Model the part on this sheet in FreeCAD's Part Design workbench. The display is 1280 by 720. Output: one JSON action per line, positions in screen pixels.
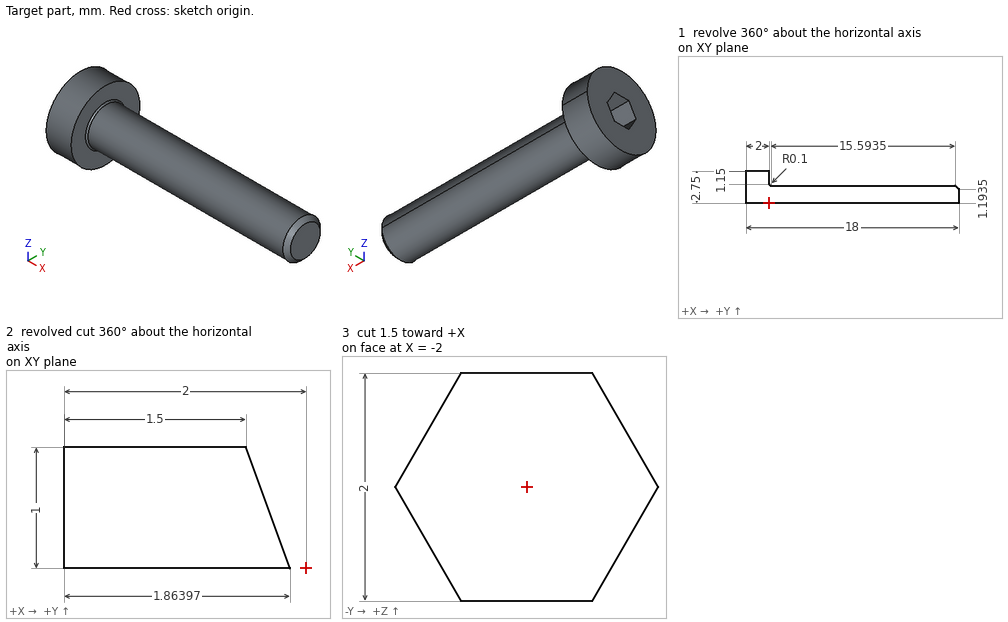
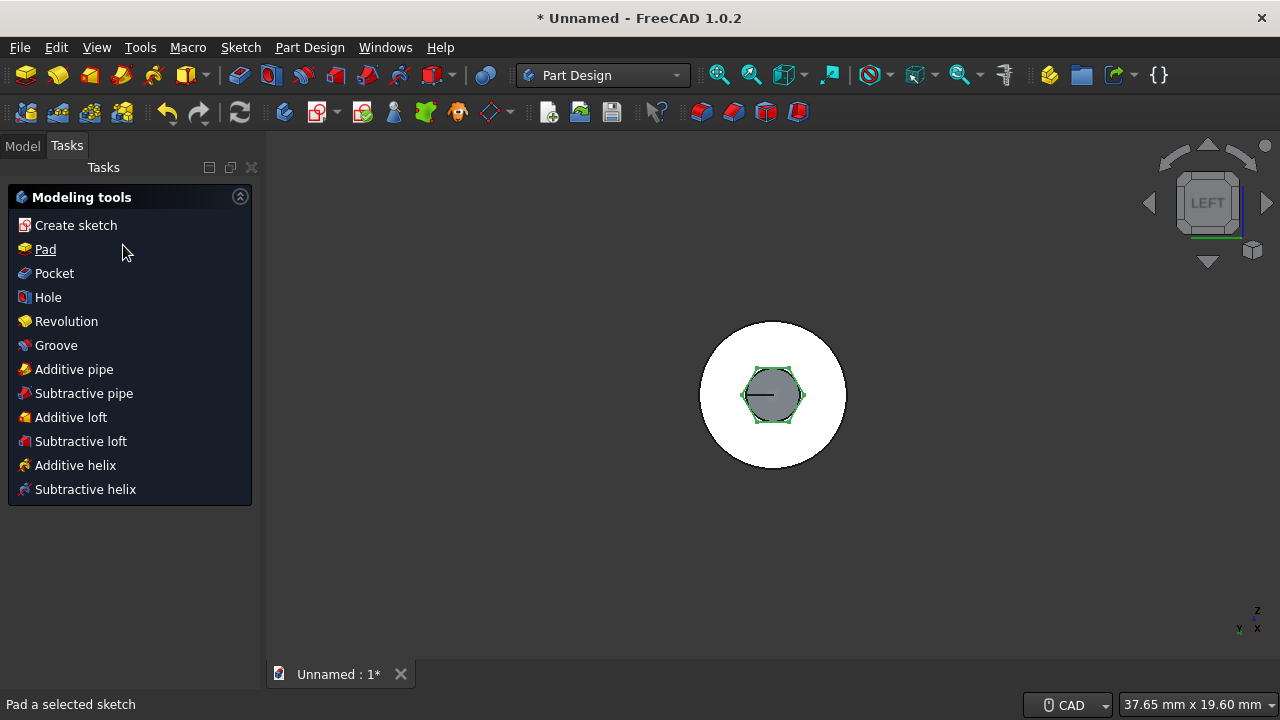
{"action": "left_click", "coordinate": [240, 76]}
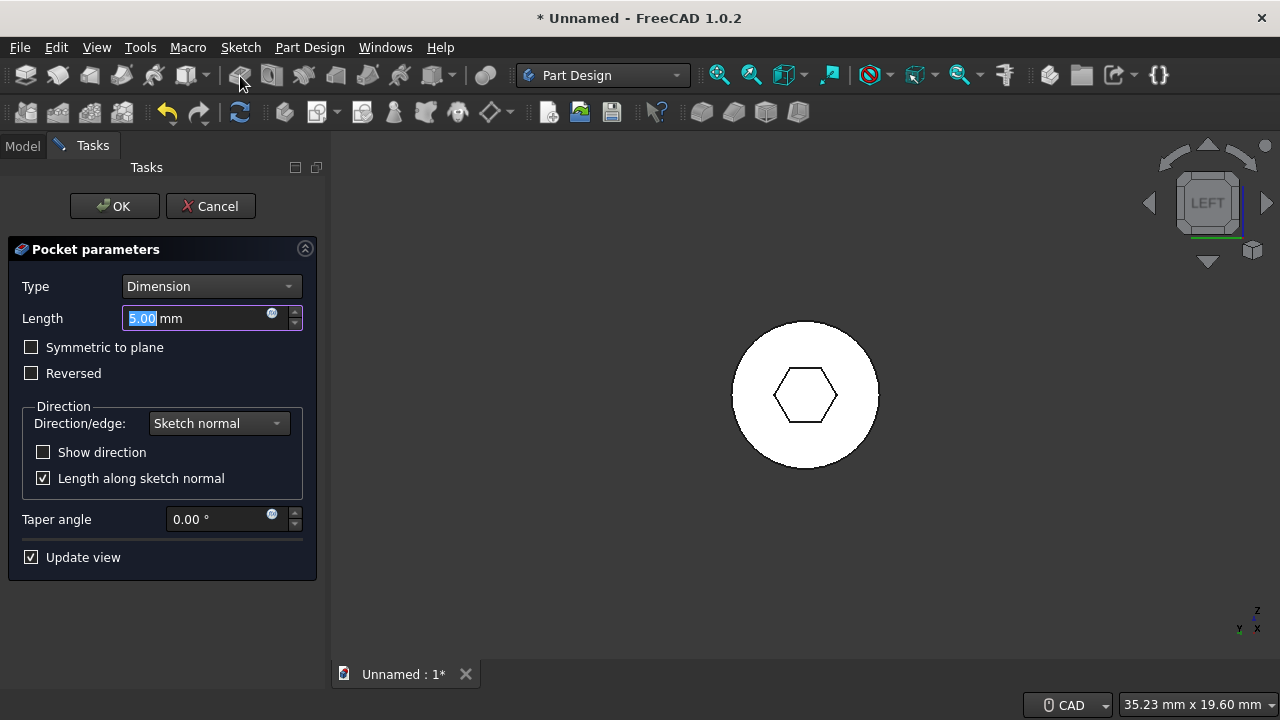
{"action": "type", "text": "1.5"}
{"action": "key", "text": "Tab"}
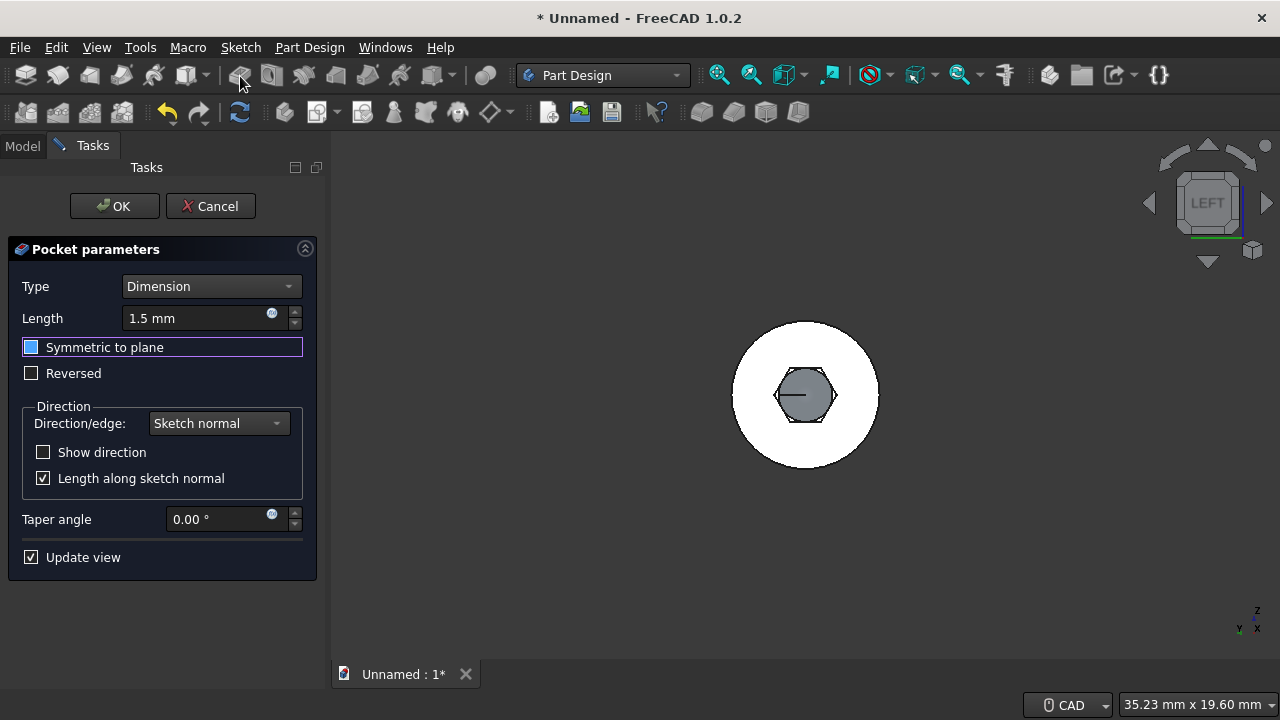
{"action": "left_click", "coordinate": [115, 206]}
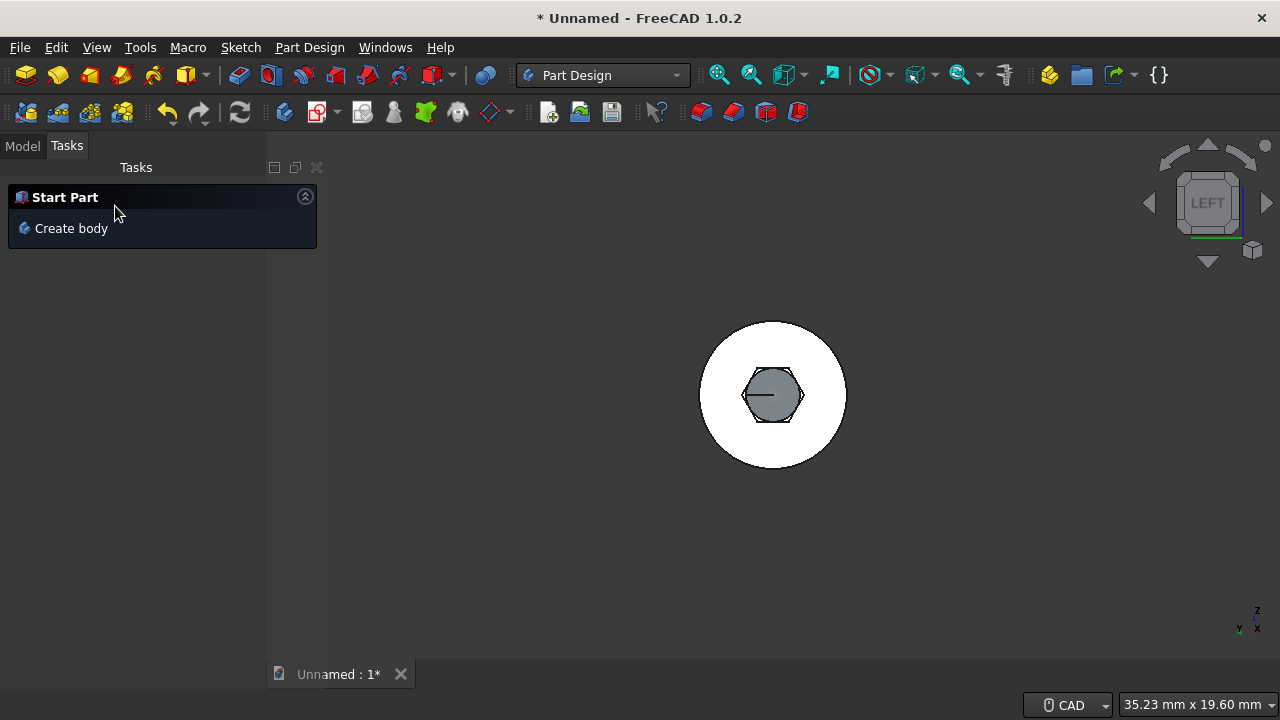
{"action": "key", "text": "0"}